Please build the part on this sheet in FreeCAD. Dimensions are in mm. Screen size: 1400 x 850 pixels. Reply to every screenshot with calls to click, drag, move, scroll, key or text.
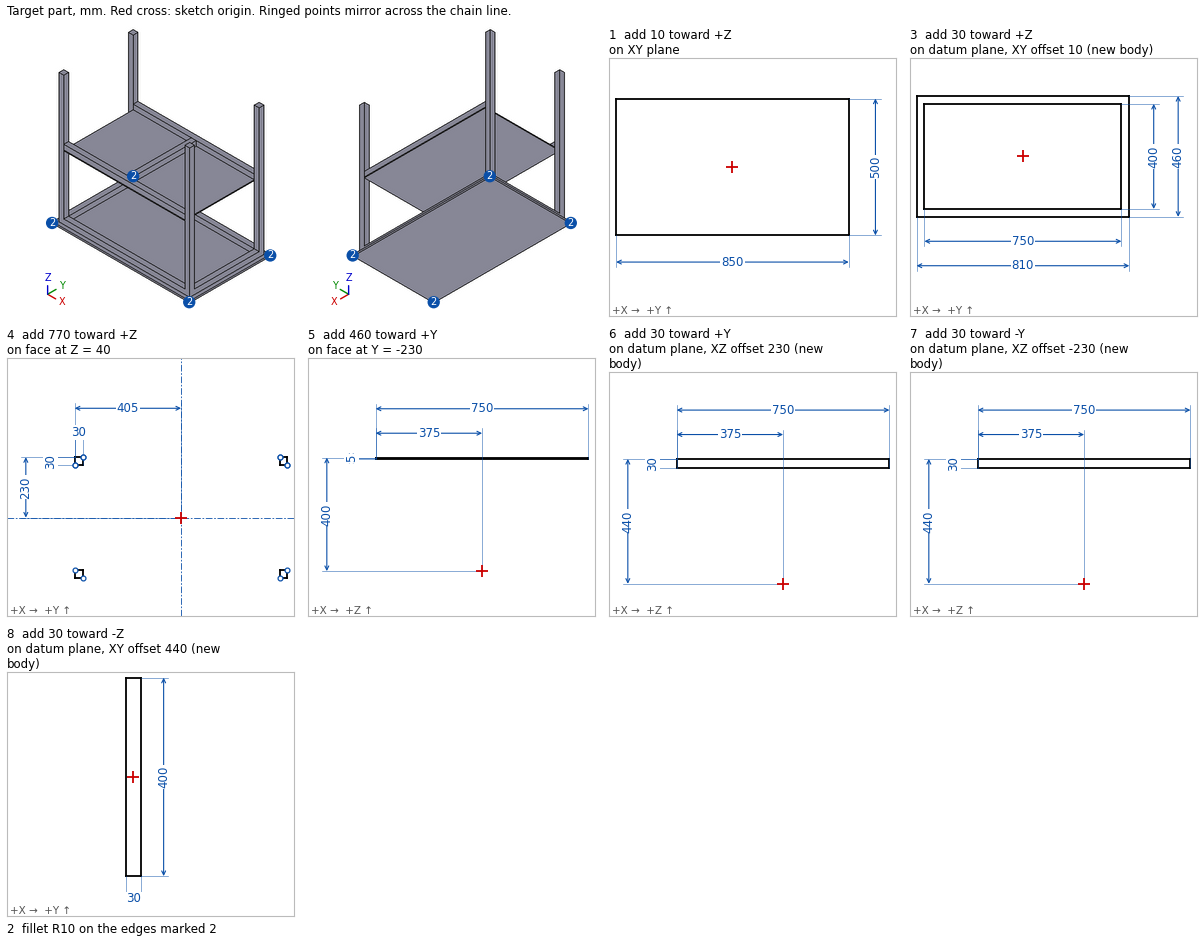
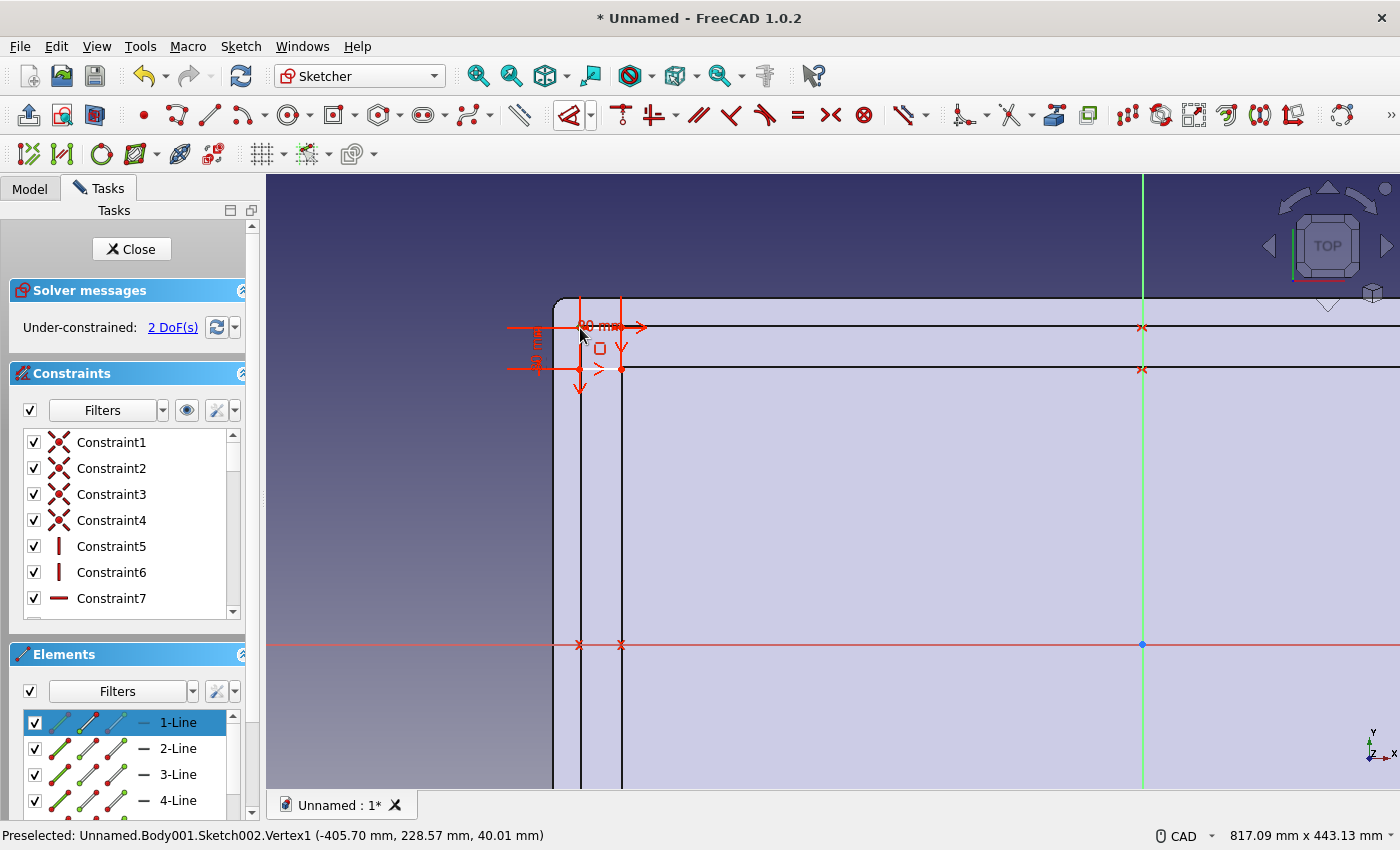
key(l)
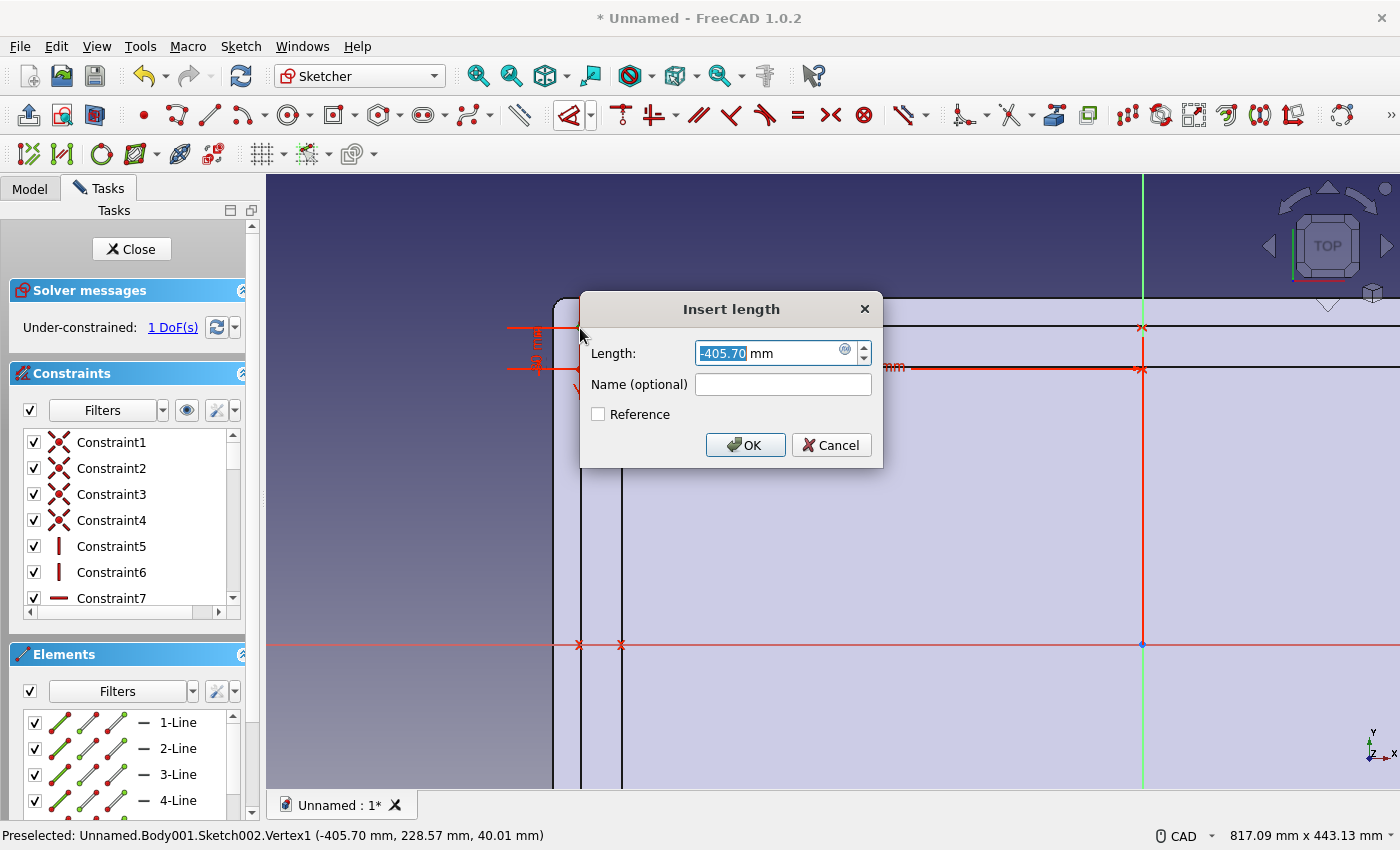
text(-405)
key(Return)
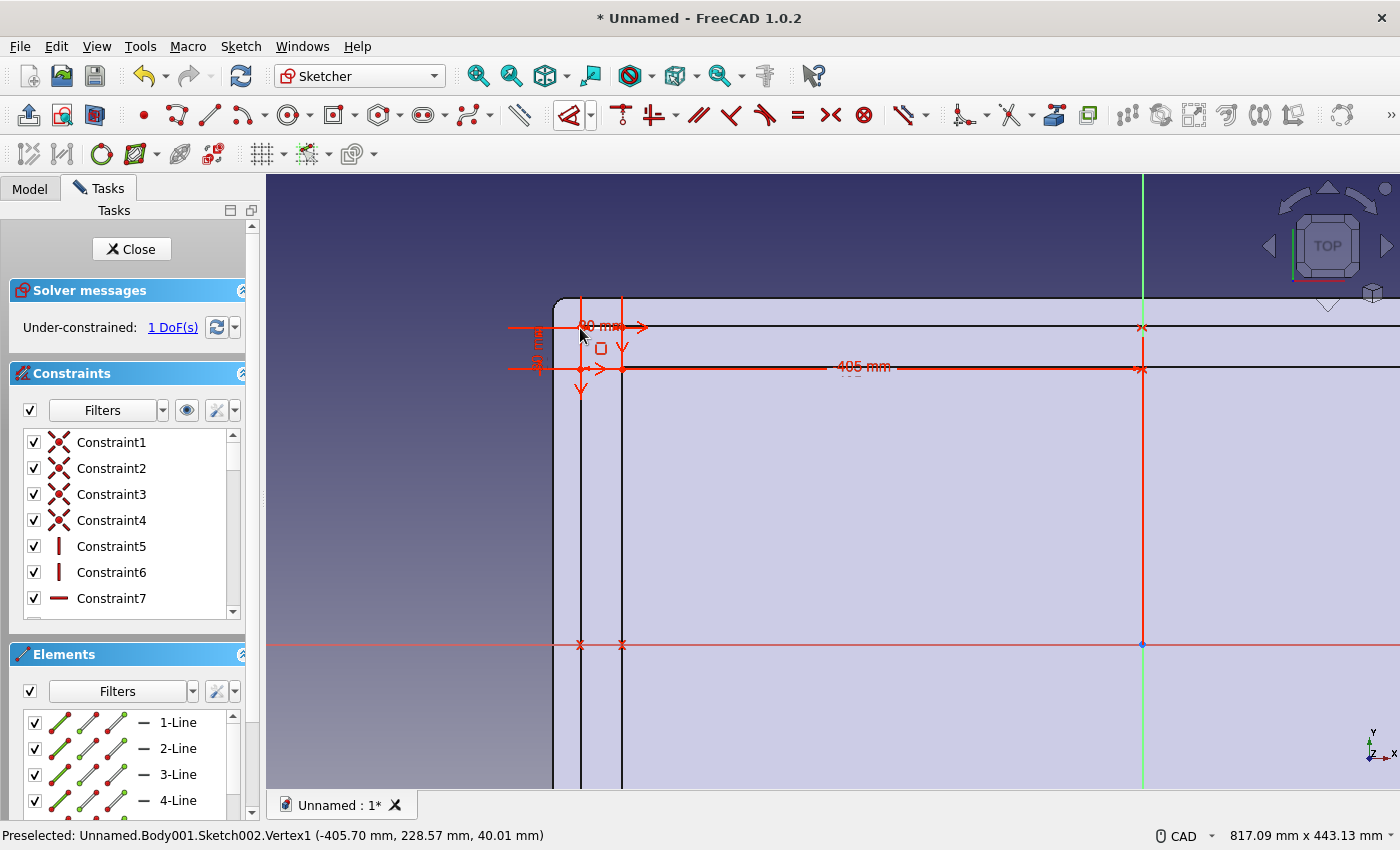
click(581, 328)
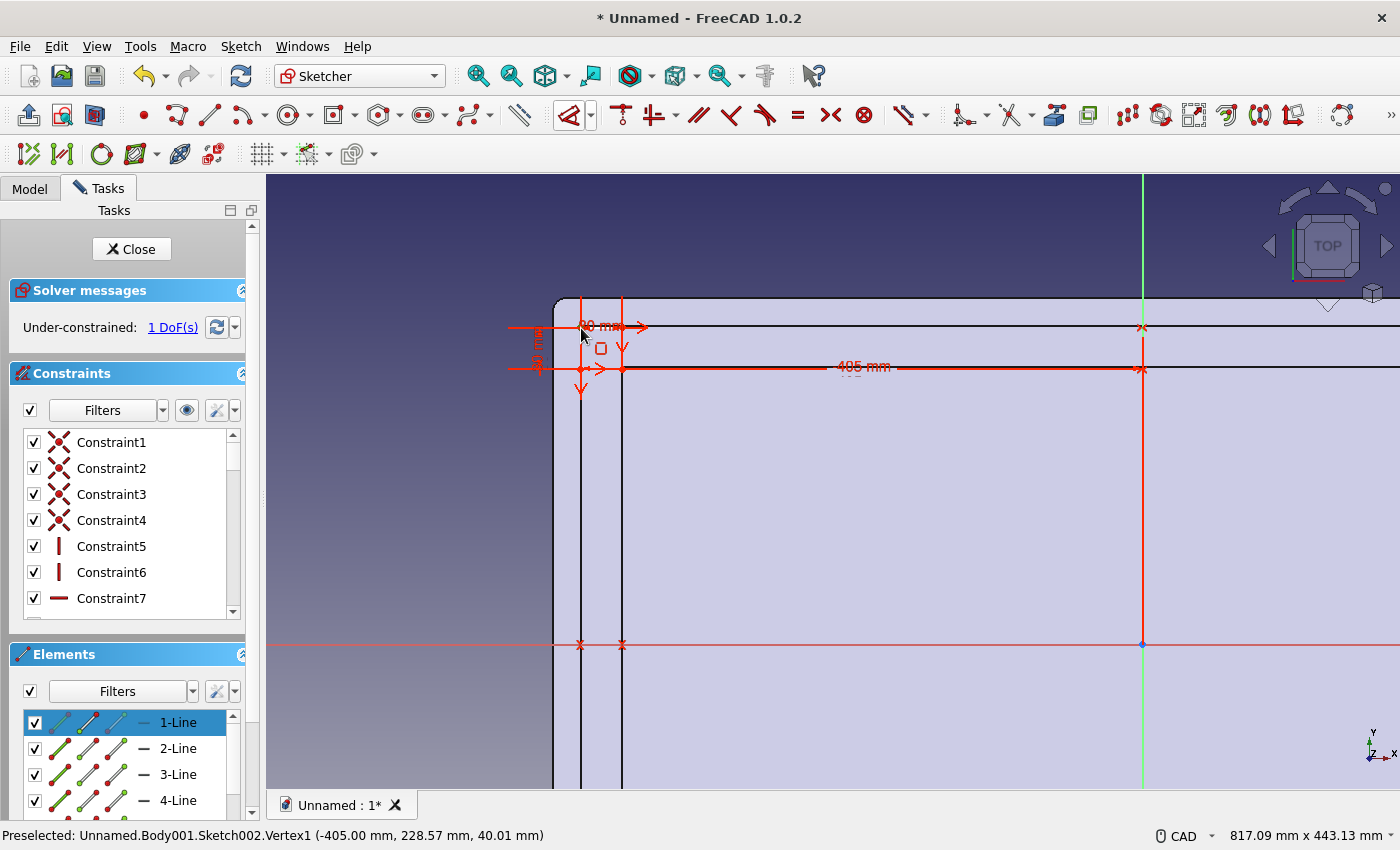
click(590, 116)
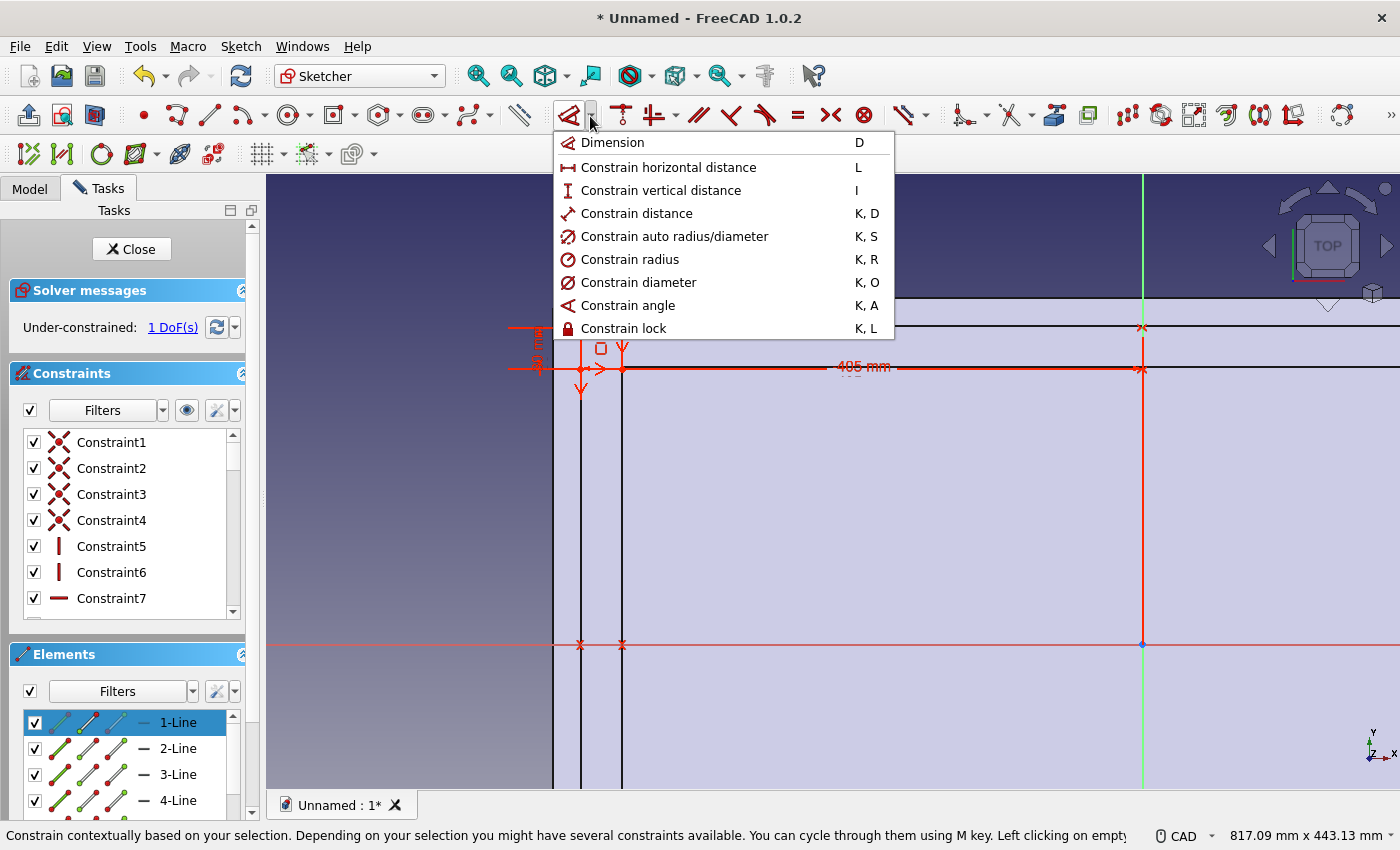
click(724, 190)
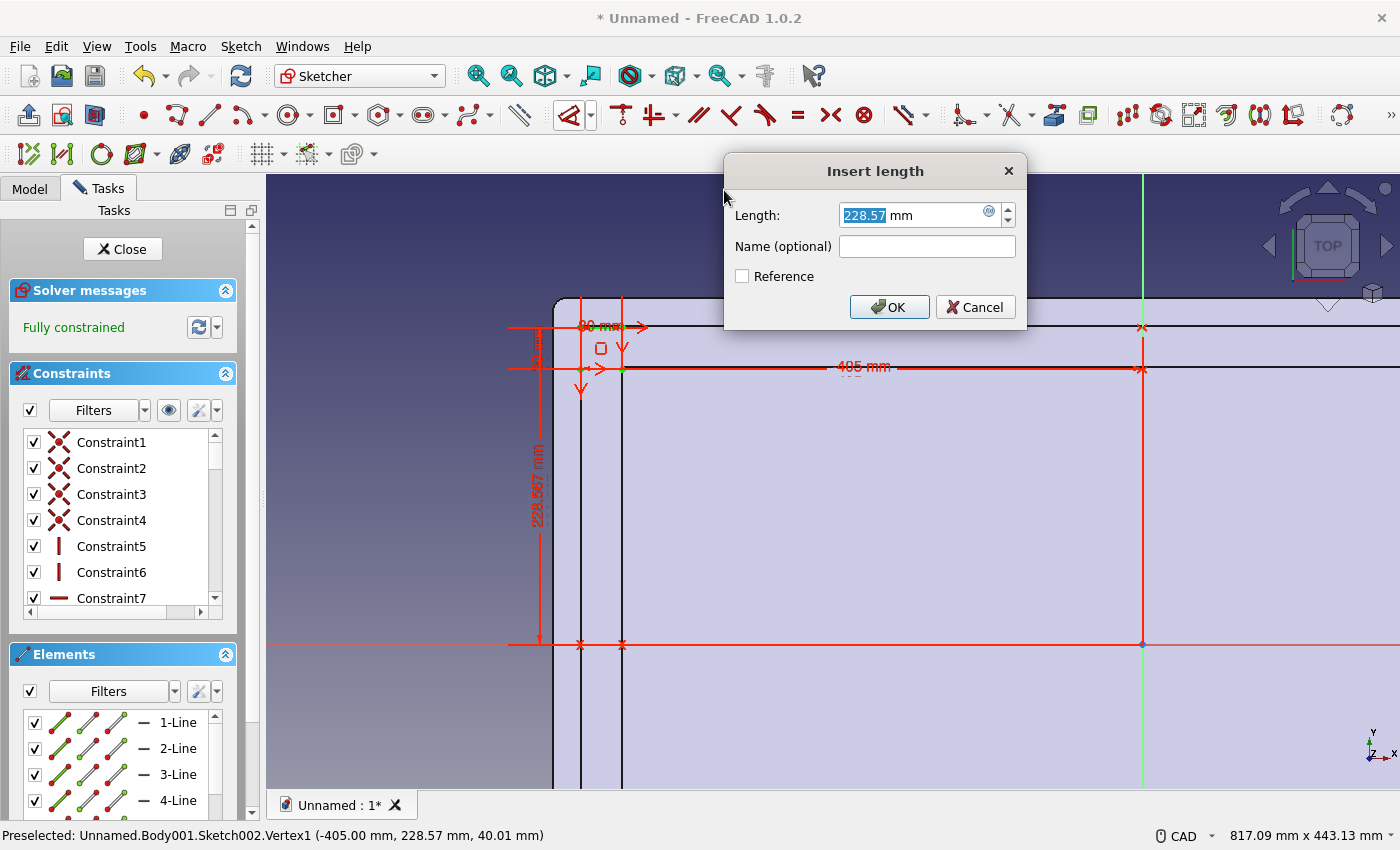
text(230)
key(Return)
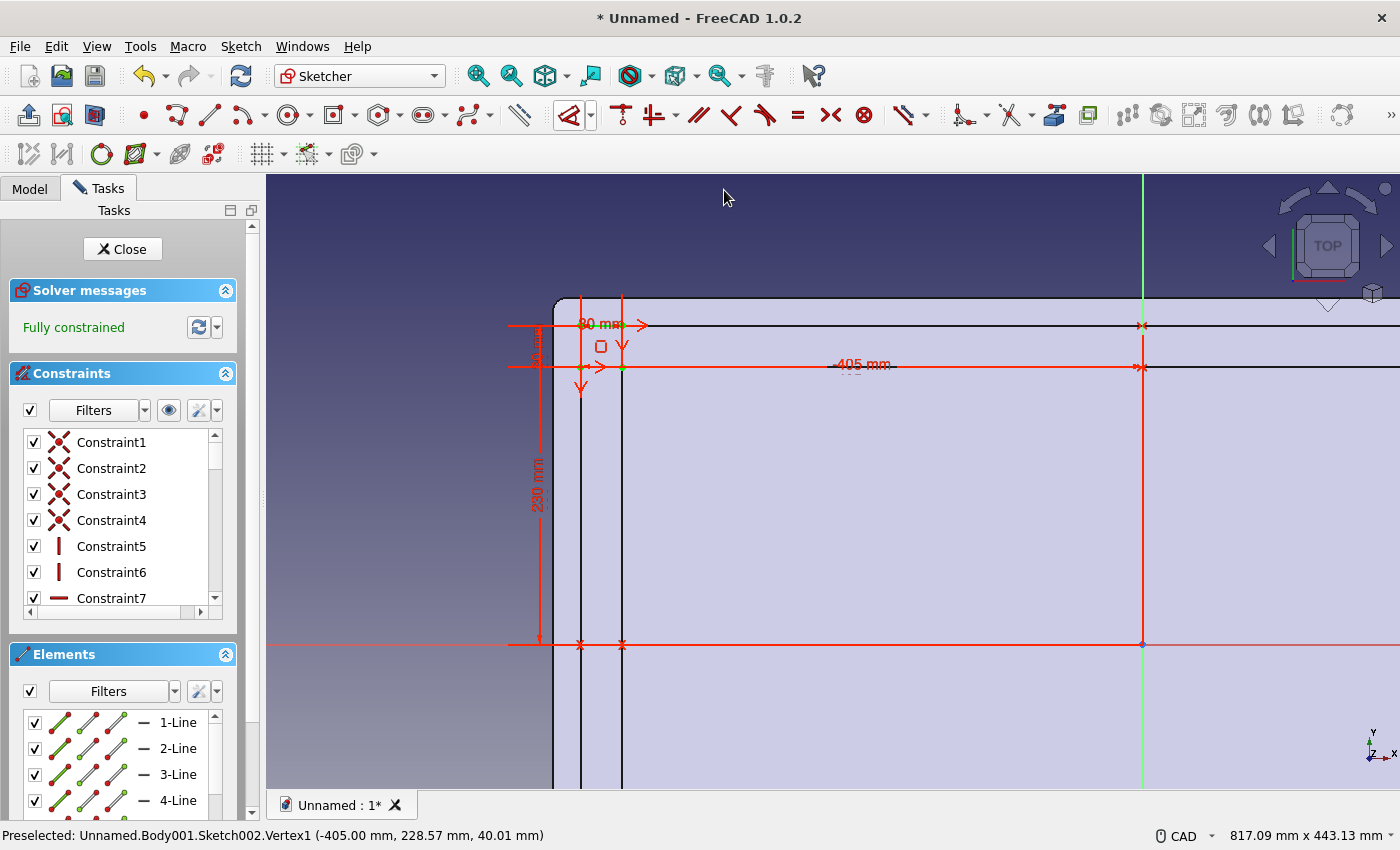
click(123, 249)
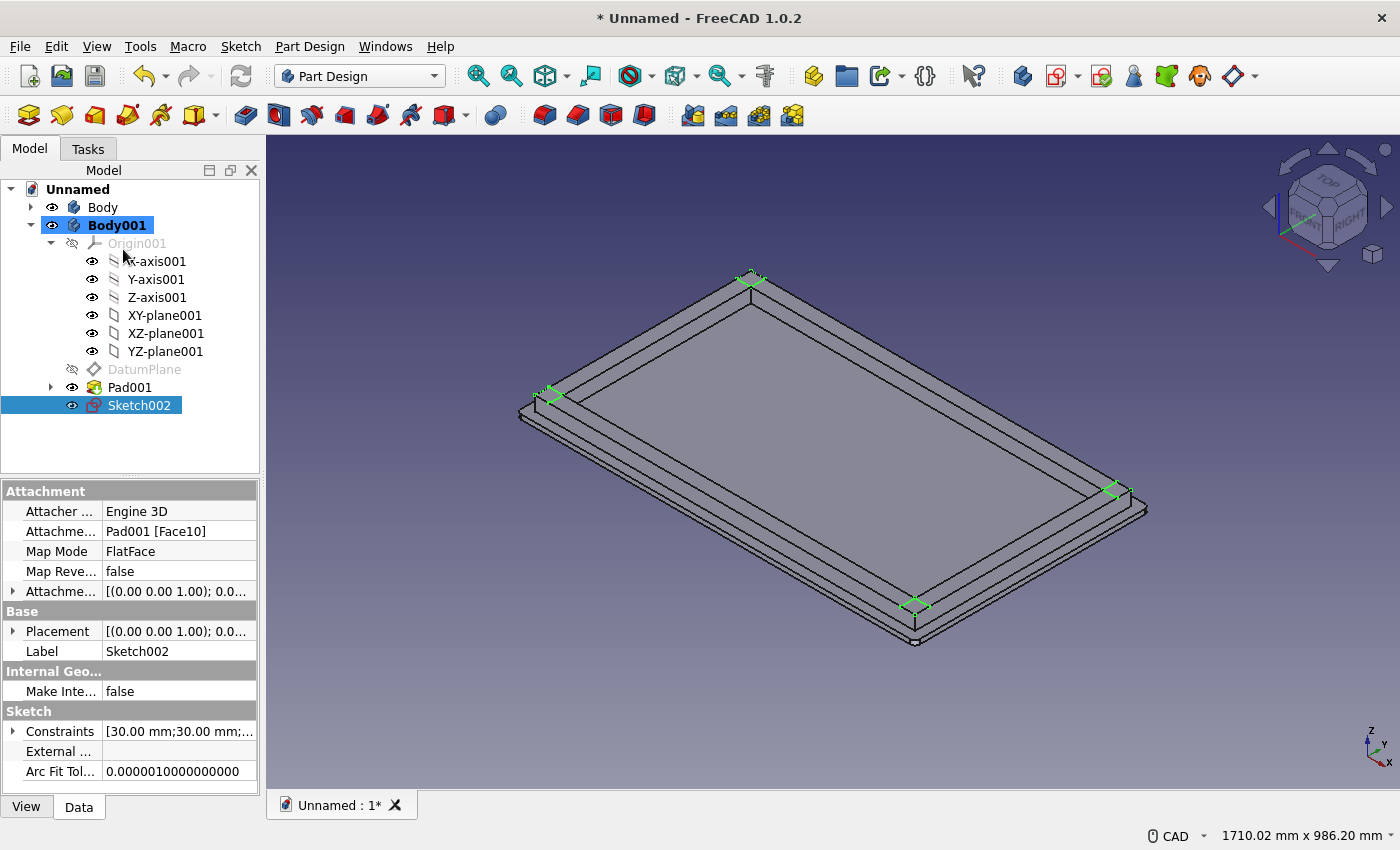
click(29, 116)